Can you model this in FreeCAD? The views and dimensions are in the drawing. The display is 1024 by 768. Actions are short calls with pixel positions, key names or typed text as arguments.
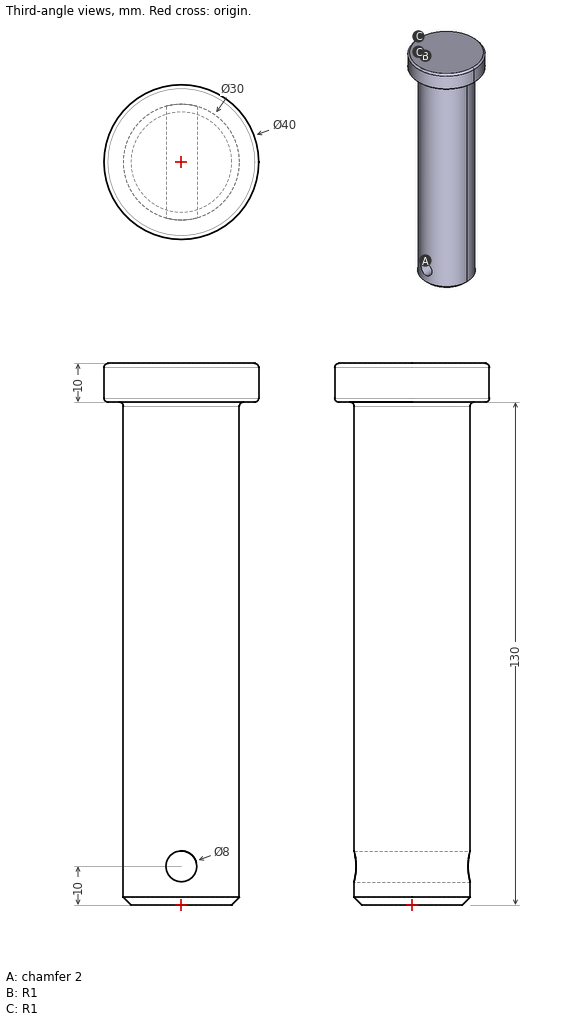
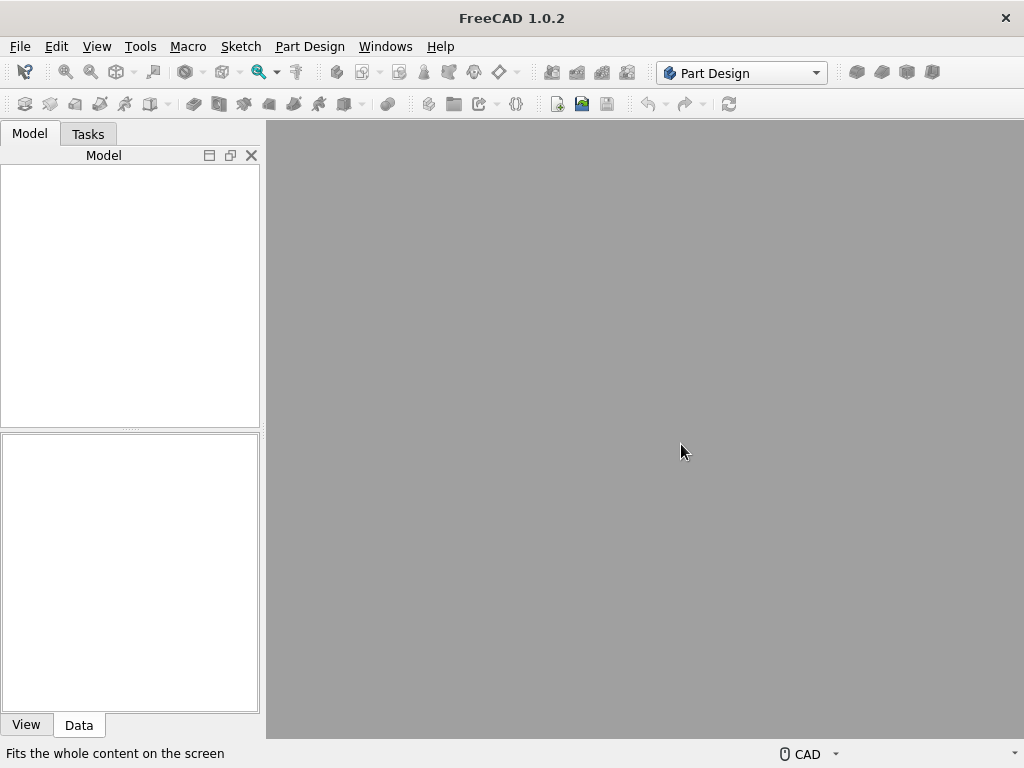
click(557, 104)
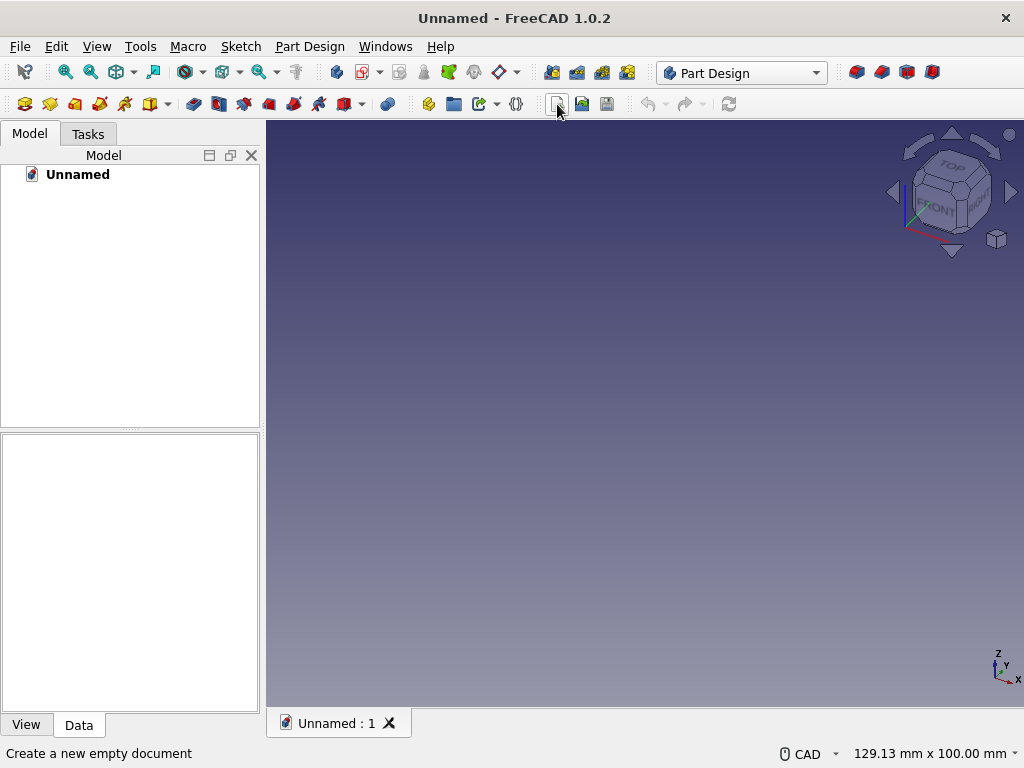
click(362, 72)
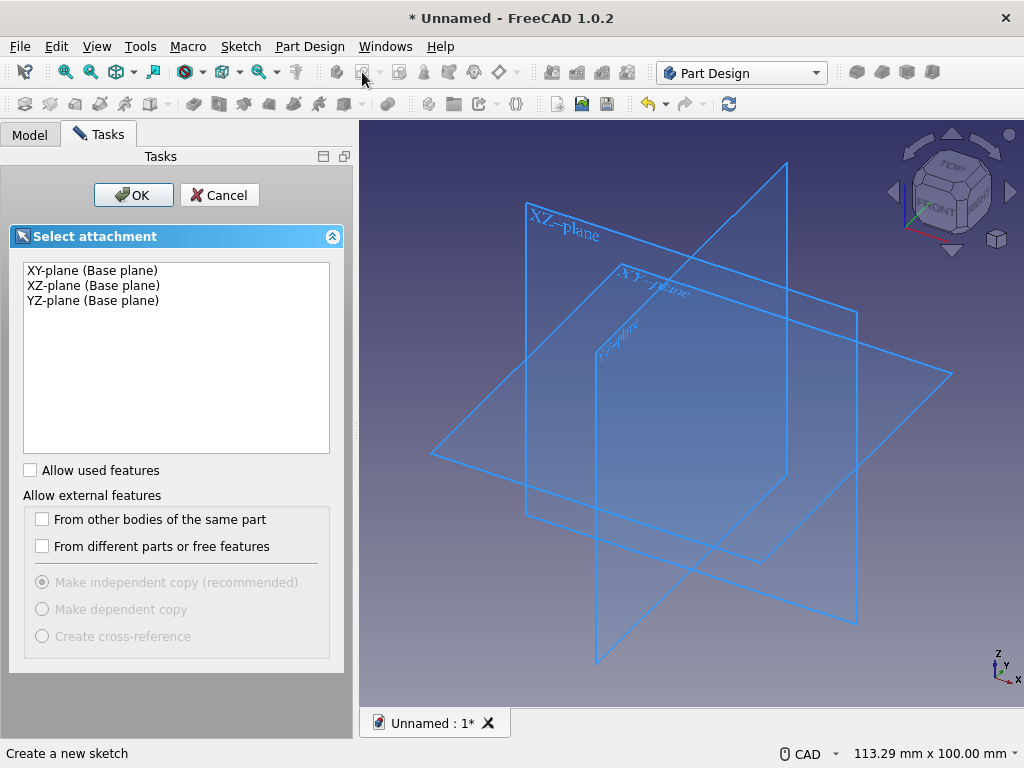
click(84, 270)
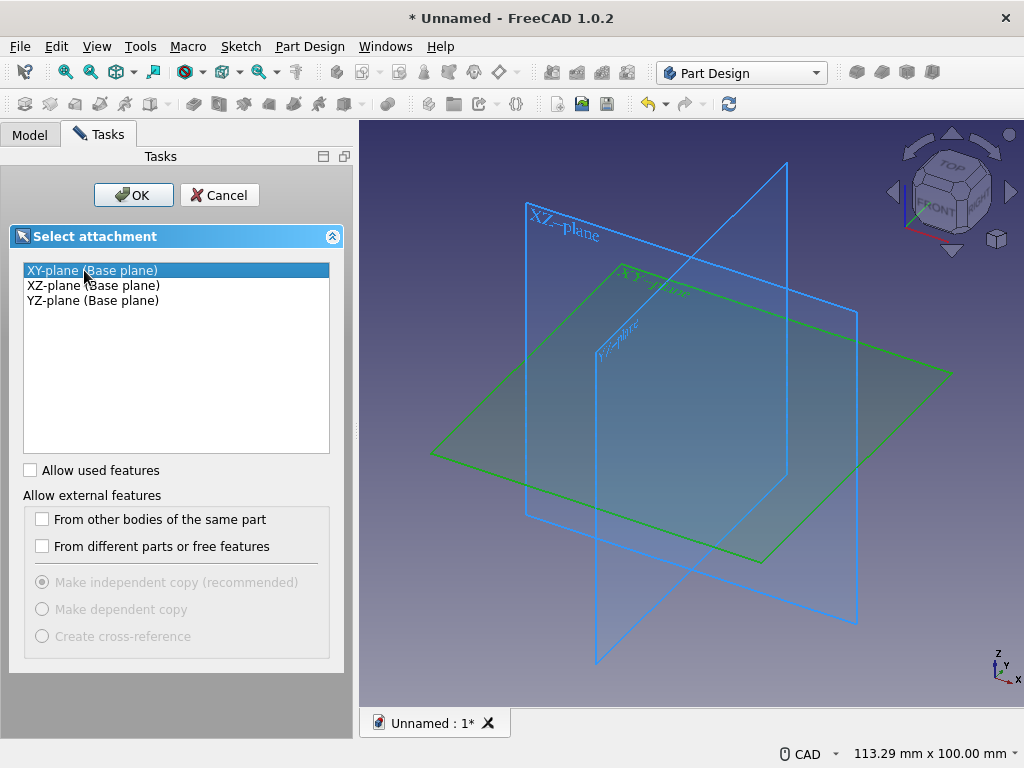
click(134, 195)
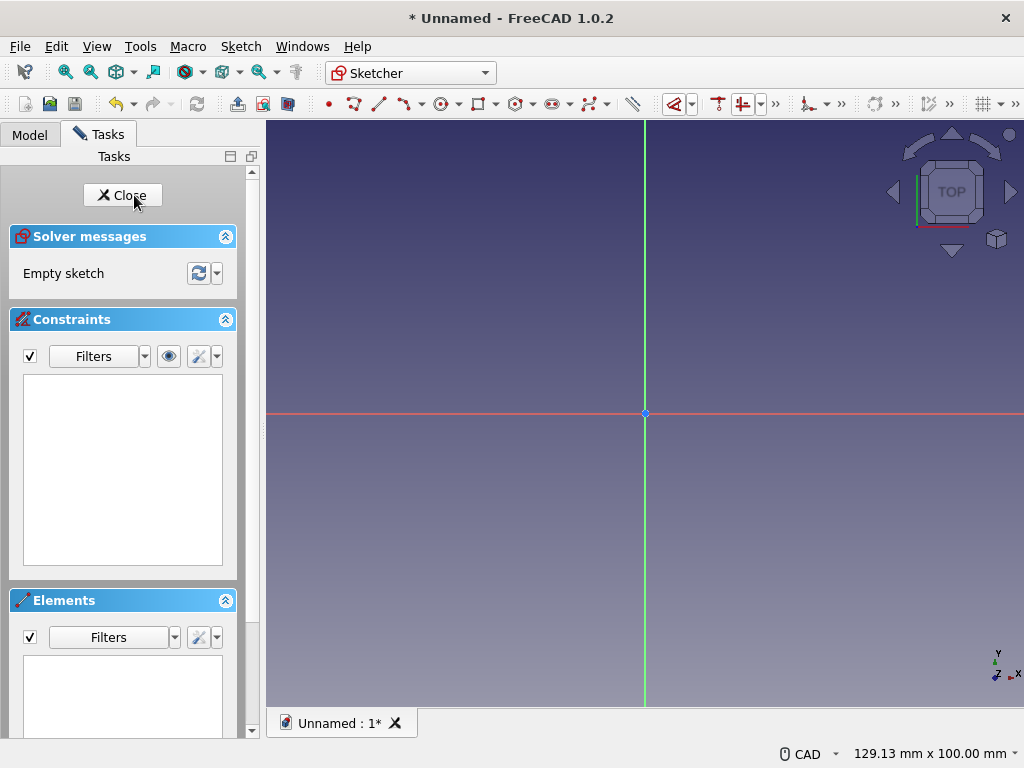
scroll(701, 413, up, 4)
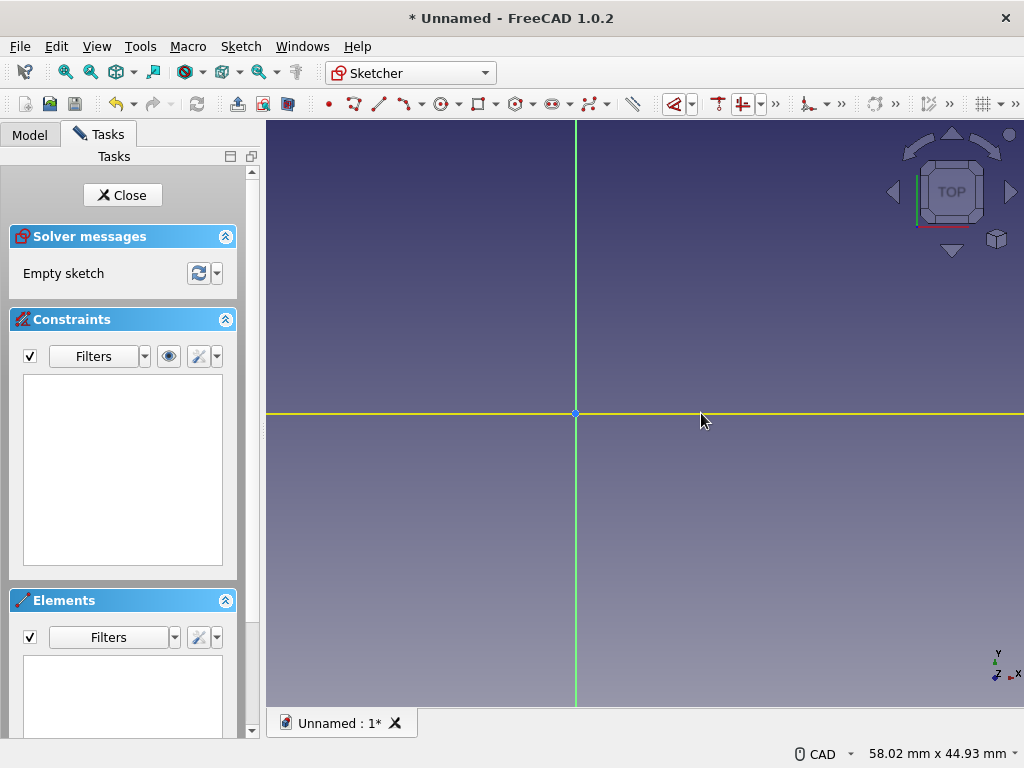
click(440, 104)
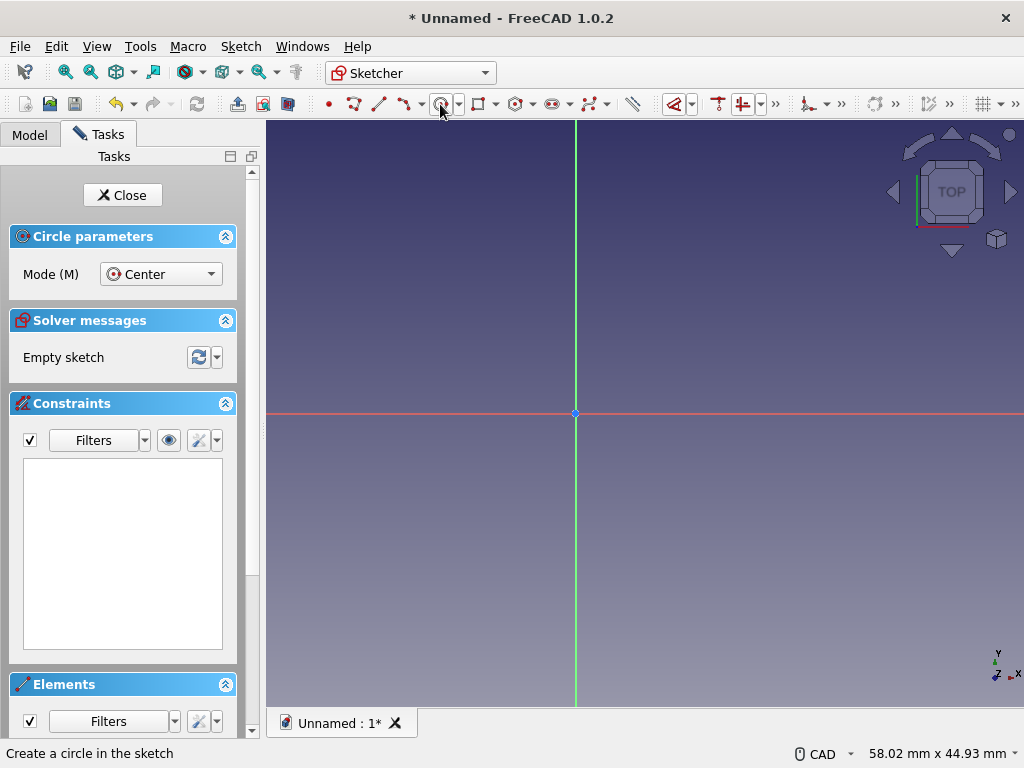
click(576, 414)
click(714, 275)
key(Escape)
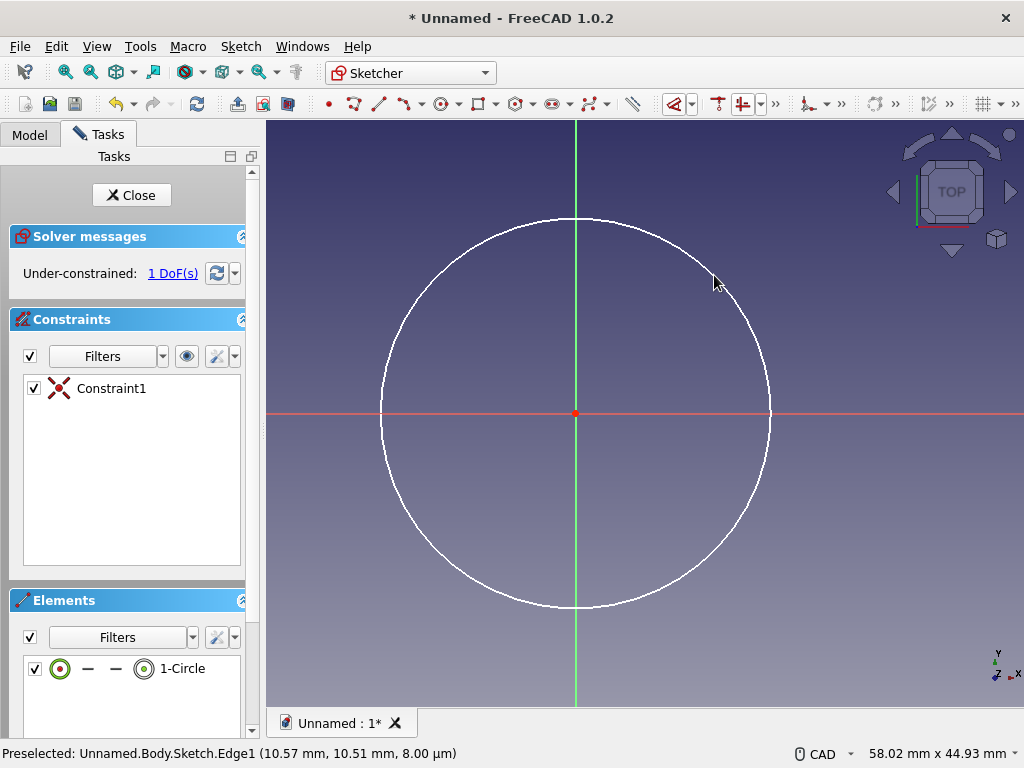
click(674, 104)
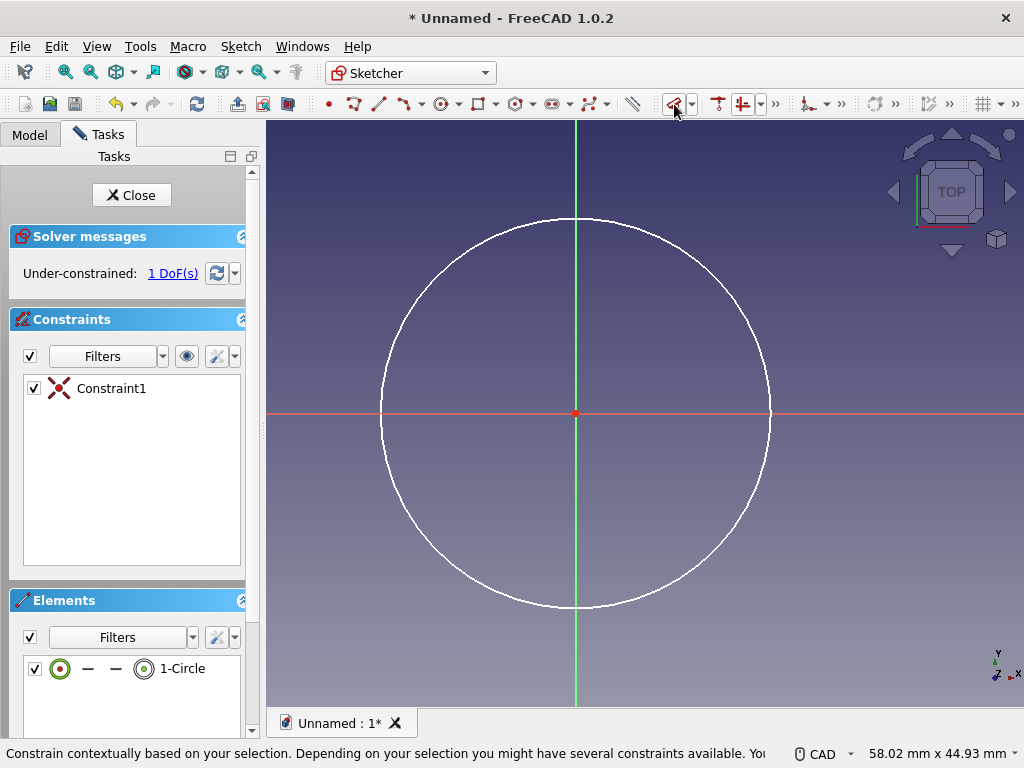
click(713, 275)
click(736, 252)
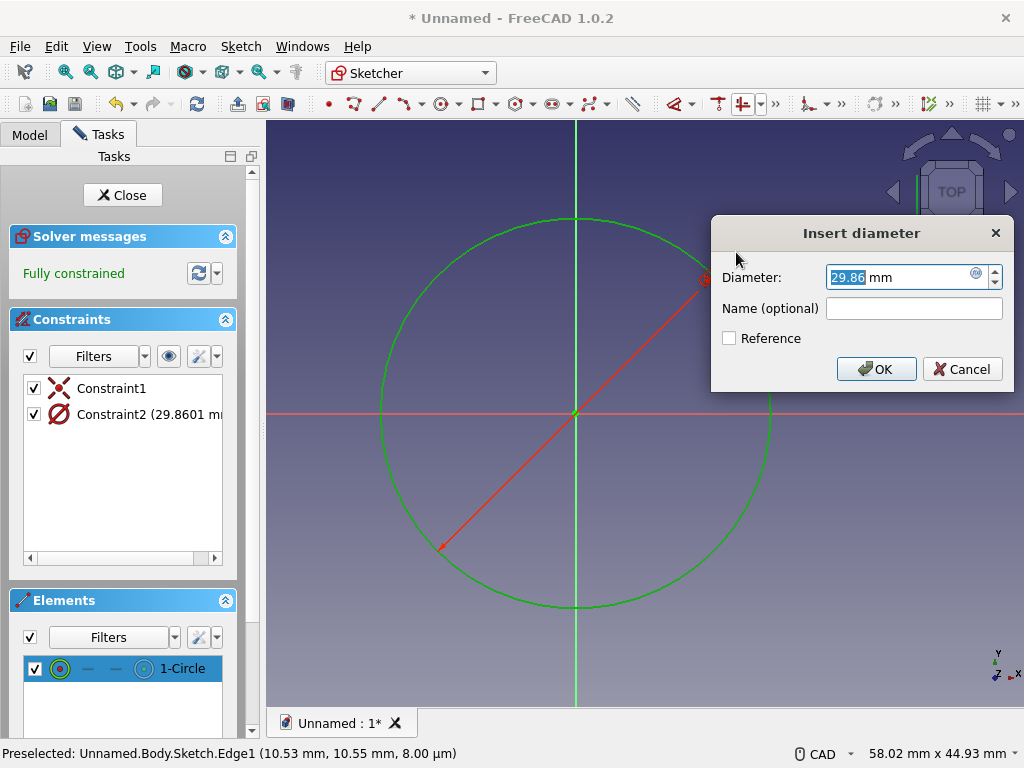
text(30)
key(Return)
key(Escape)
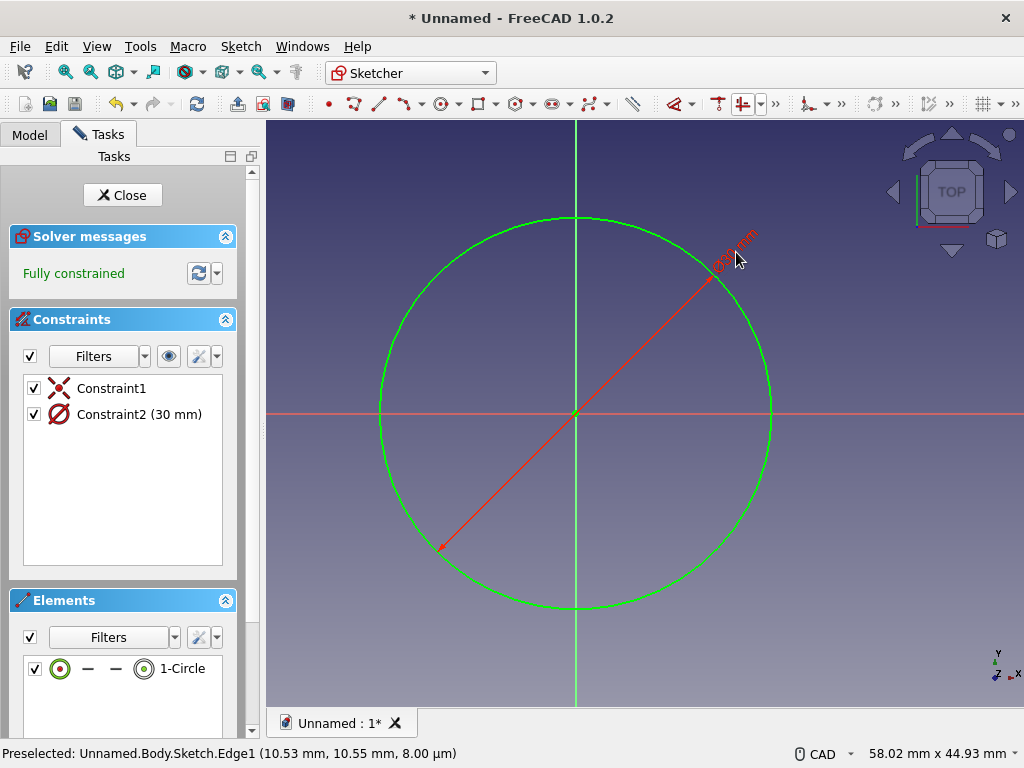
click(123, 195)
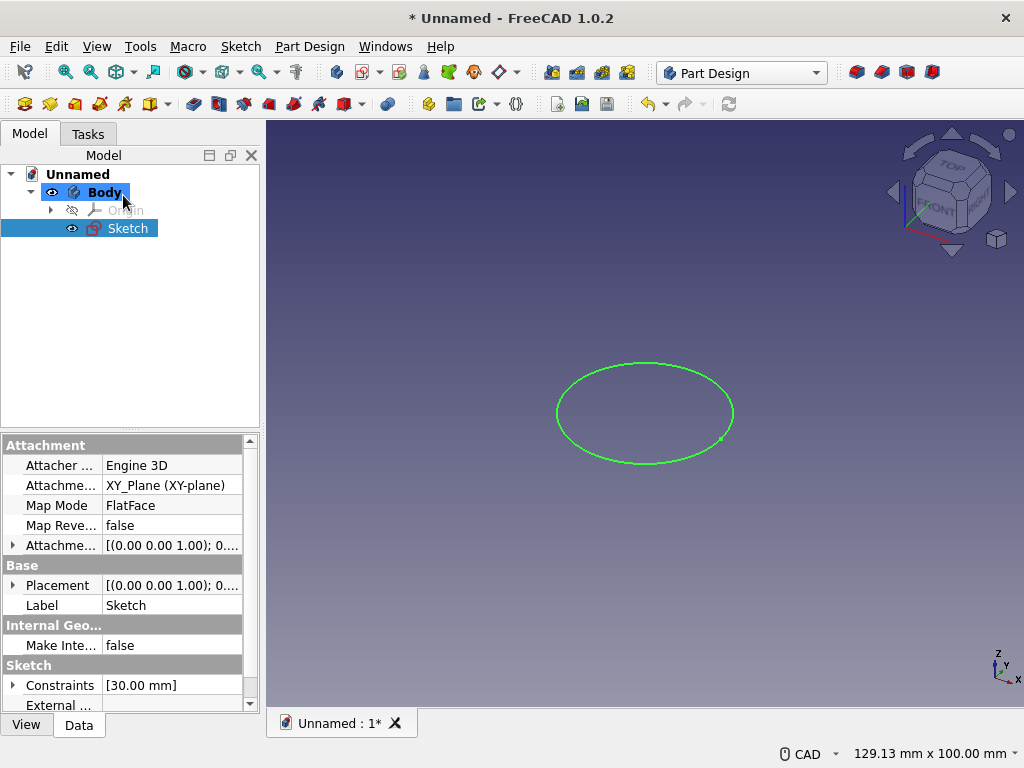
click(25, 104)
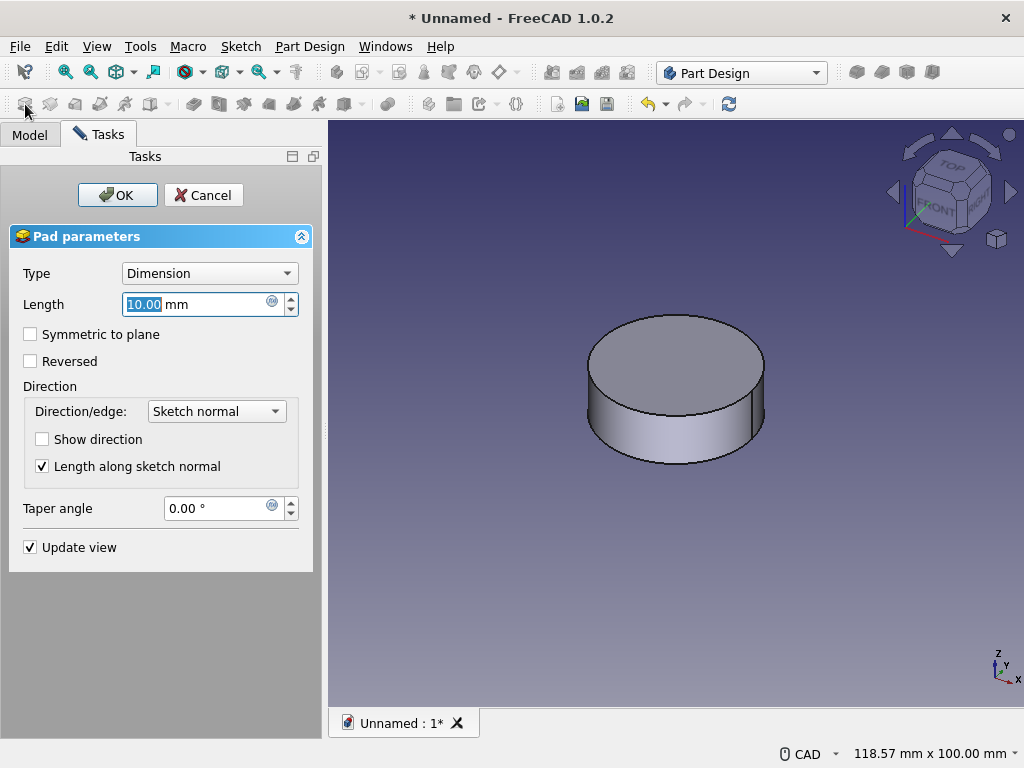
text(130)
key(Tab)